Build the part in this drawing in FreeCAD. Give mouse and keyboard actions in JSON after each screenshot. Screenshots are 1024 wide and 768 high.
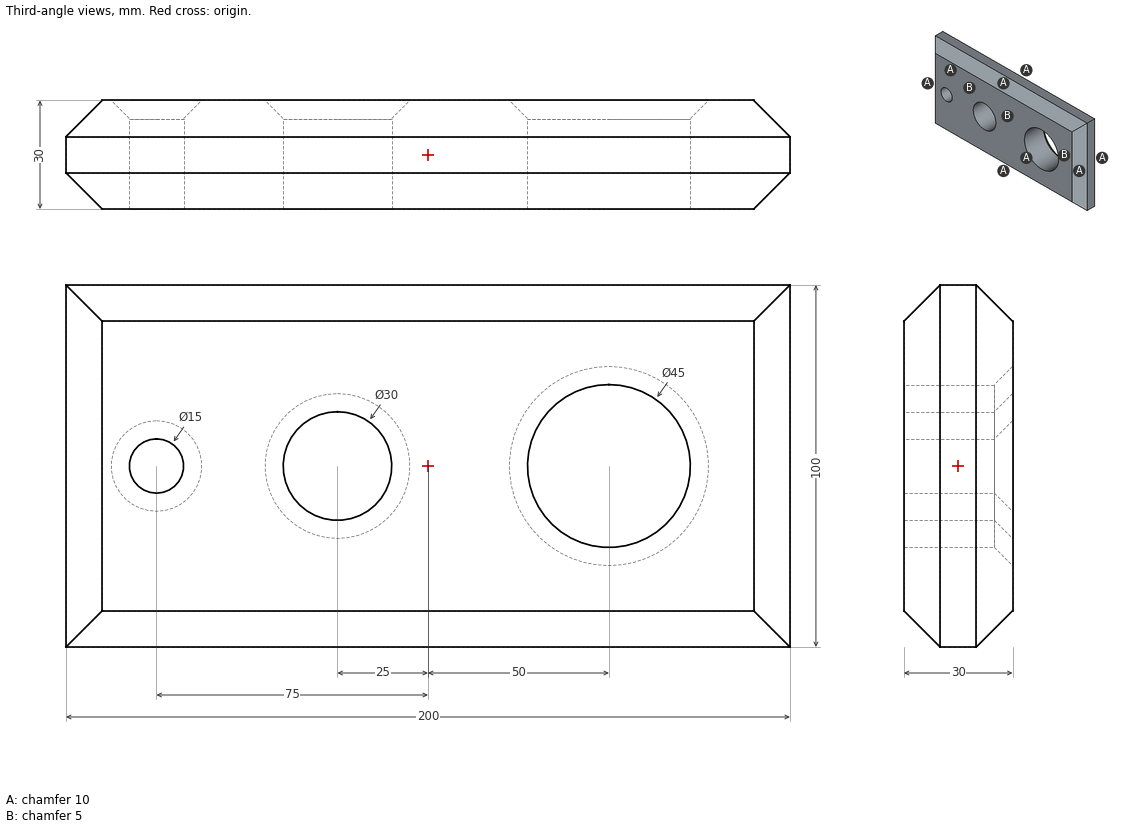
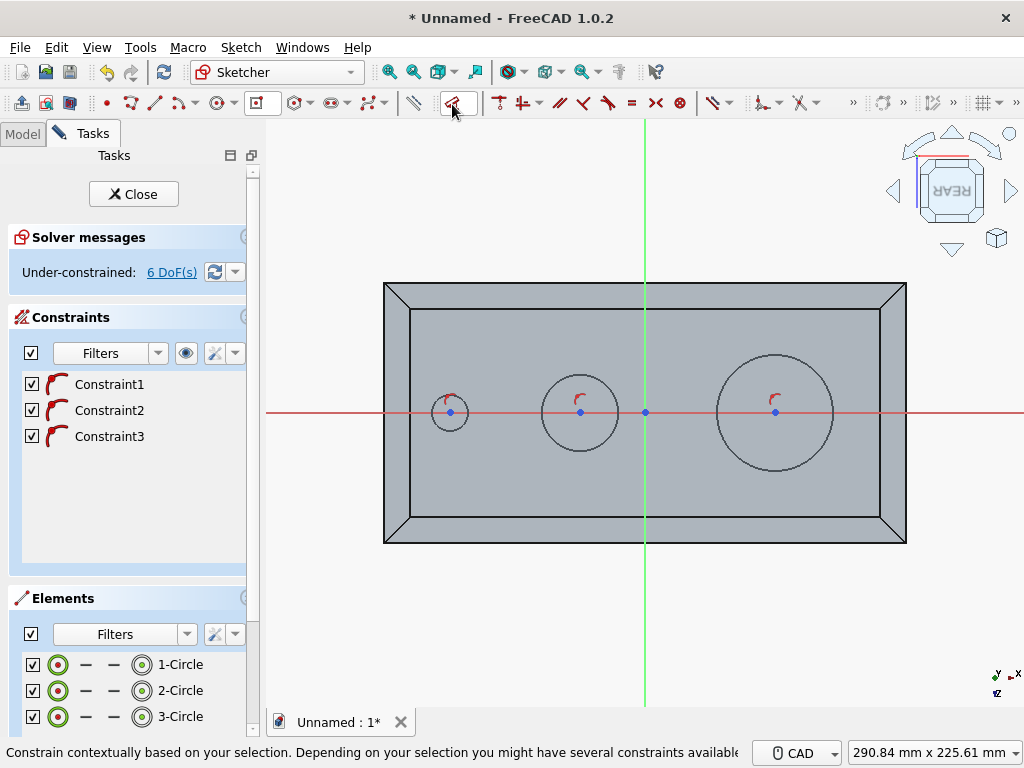
{"action": "left_click", "coordinate": [463, 400]}
{"action": "left_click", "coordinate": [486, 377]}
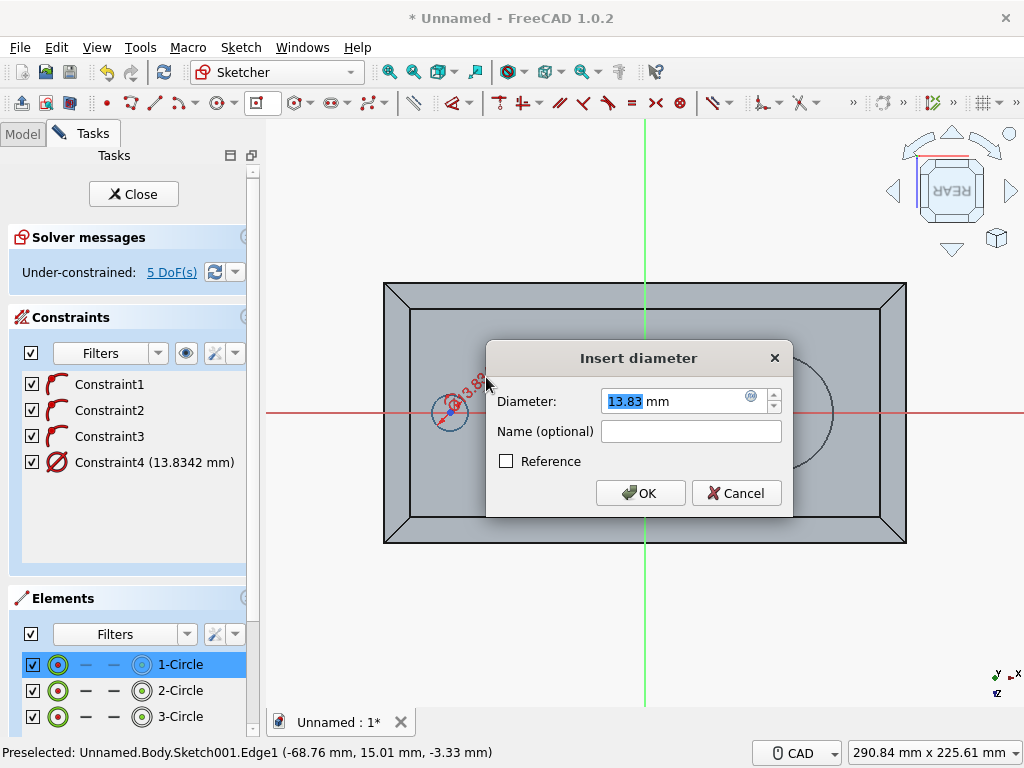
{"action": "type", "text": "15"}
{"action": "key", "text": "Return"}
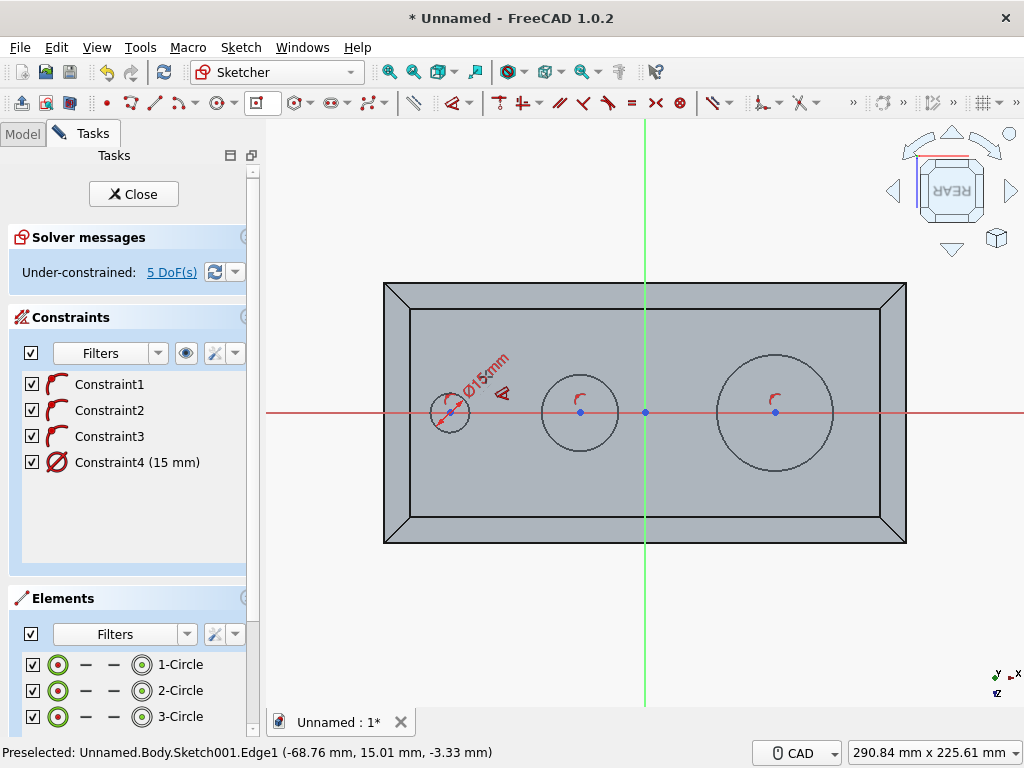
{"action": "left_click", "coordinate": [607, 386]}
{"action": "left_click", "coordinate": [630, 363]}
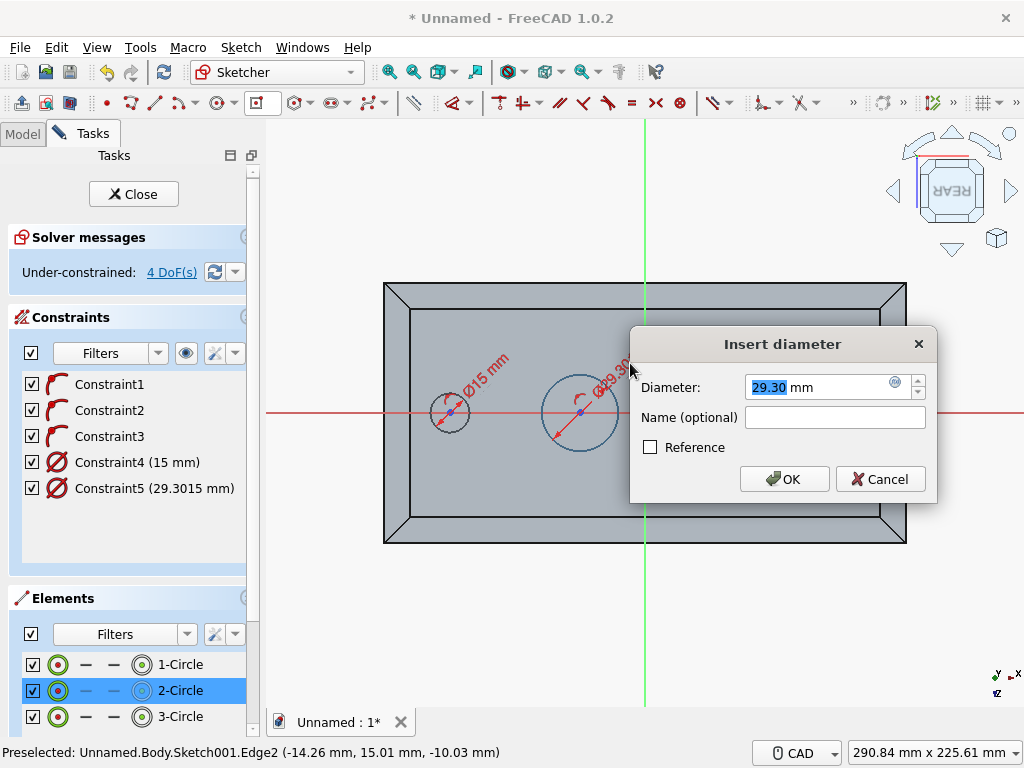
{"action": "type", "text": "30"}
{"action": "key", "text": "Return"}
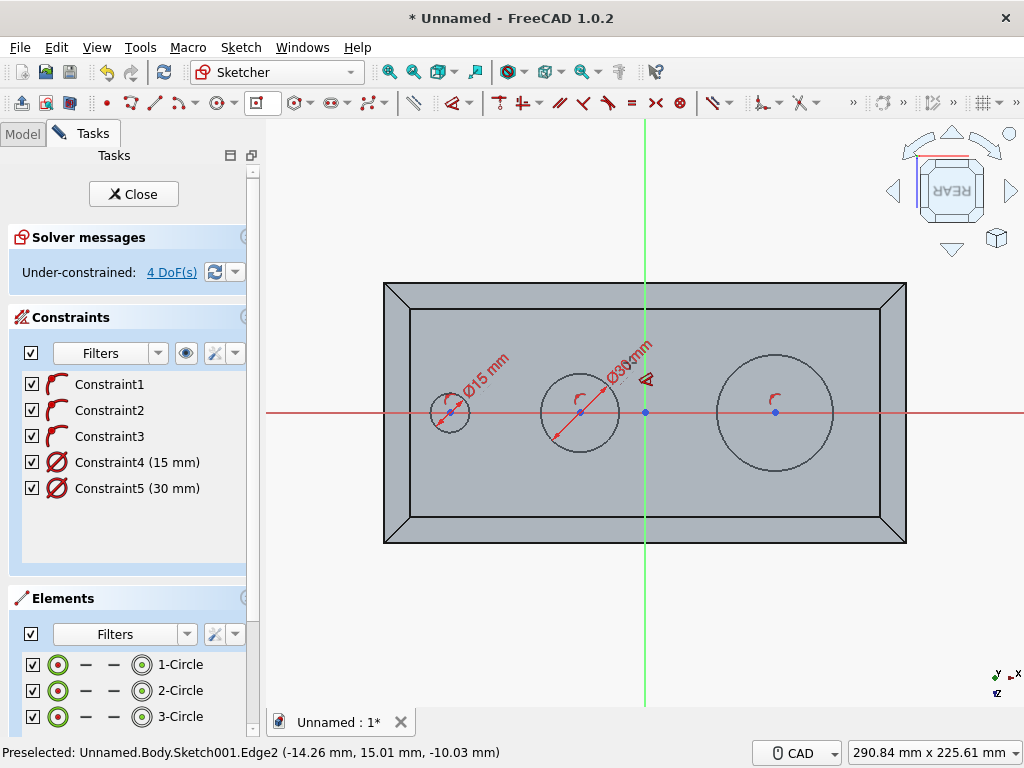
{"action": "left_click", "coordinate": [816, 372]}
{"action": "left_click", "coordinate": [839, 349]}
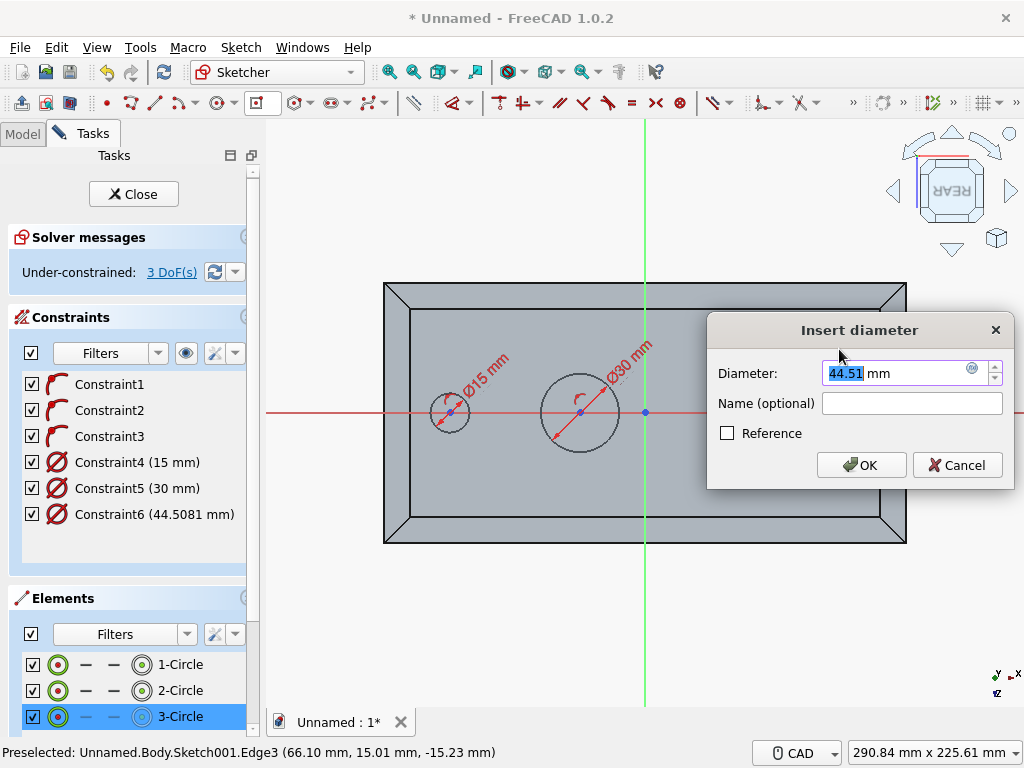
{"action": "type", "text": "45"}
{"action": "key", "text": "Return"}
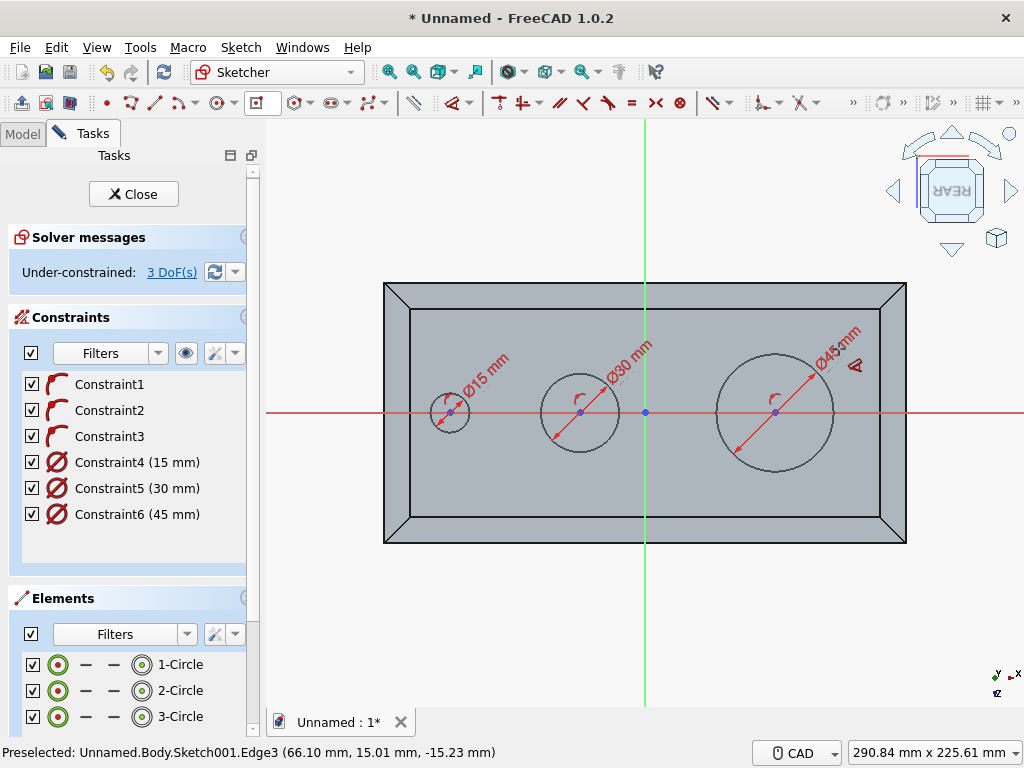
{"action": "left_click", "coordinate": [450, 413]}
{"action": "left_click", "coordinate": [503, 447]}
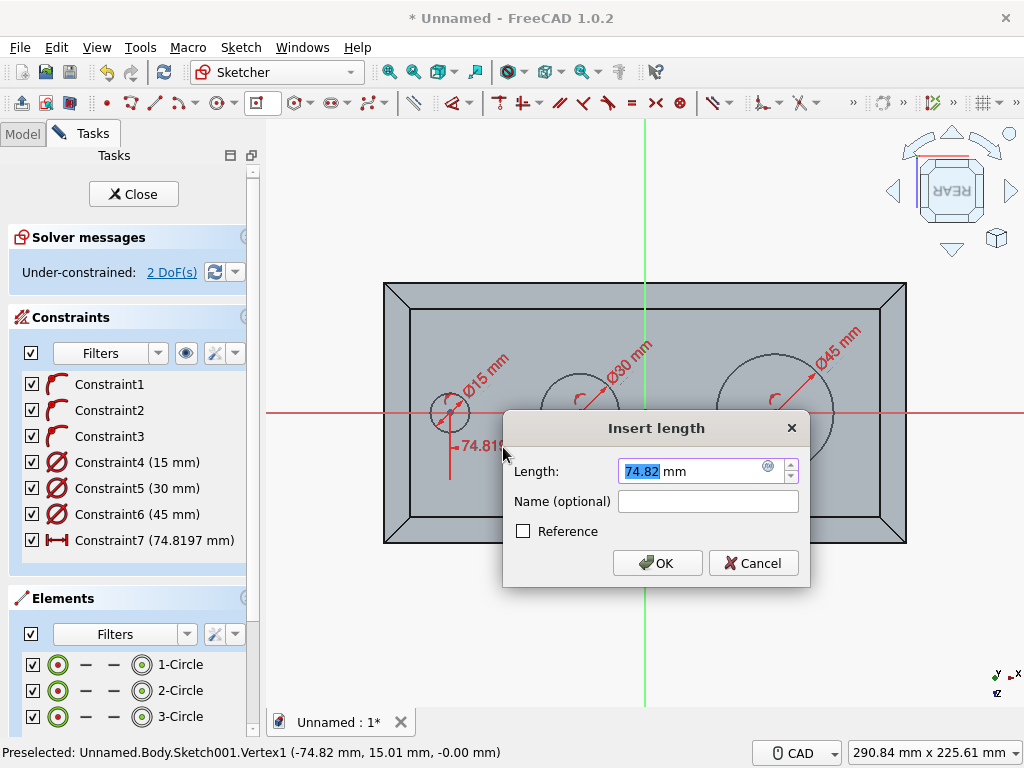
{"action": "type", "text": "75"}
{"action": "key", "text": "Return"}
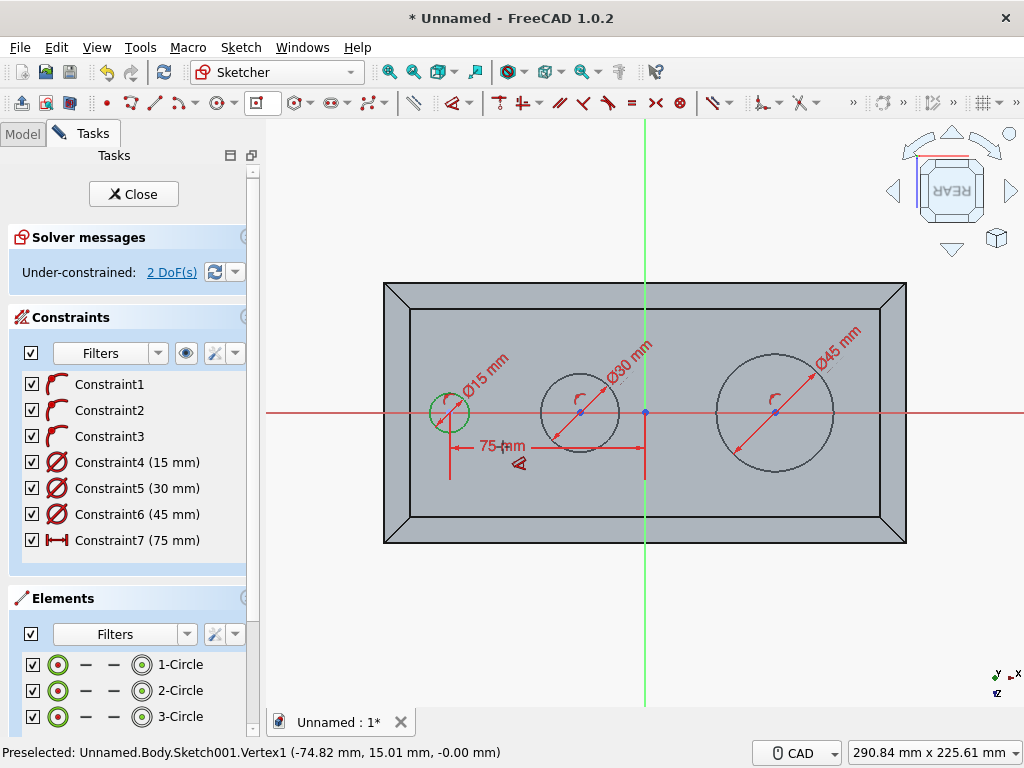
{"action": "left_click", "coordinate": [580, 413]}
{"action": "left_click", "coordinate": [627, 447]}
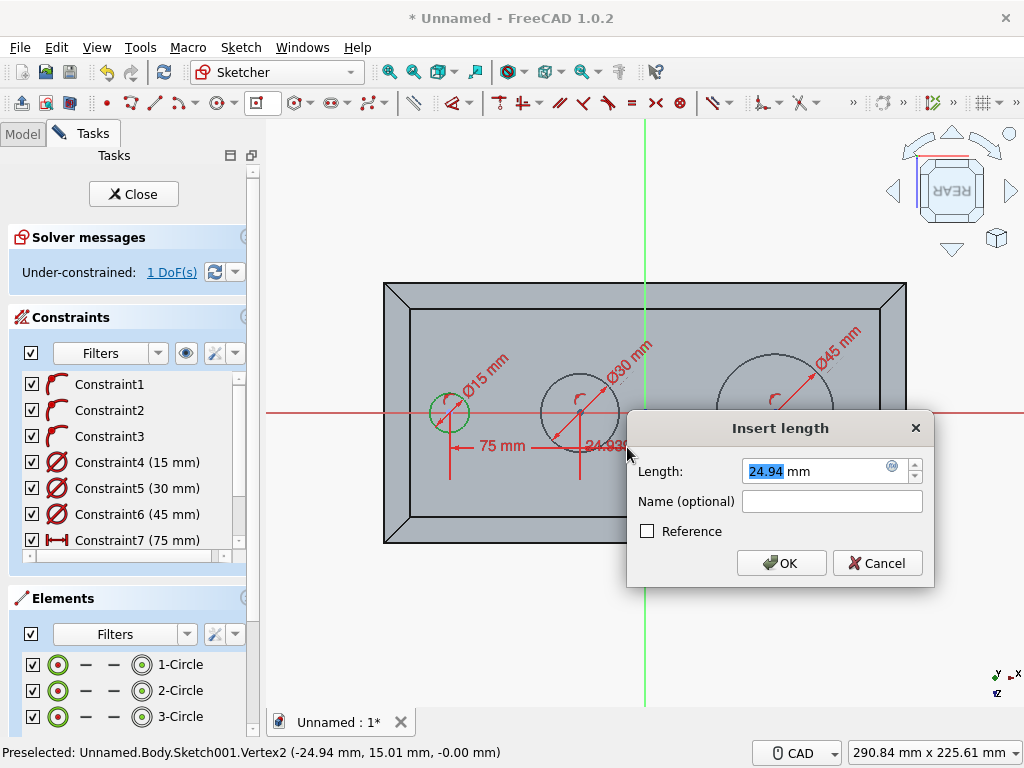
{"action": "type", "text": "25"}
{"action": "key", "text": "Return"}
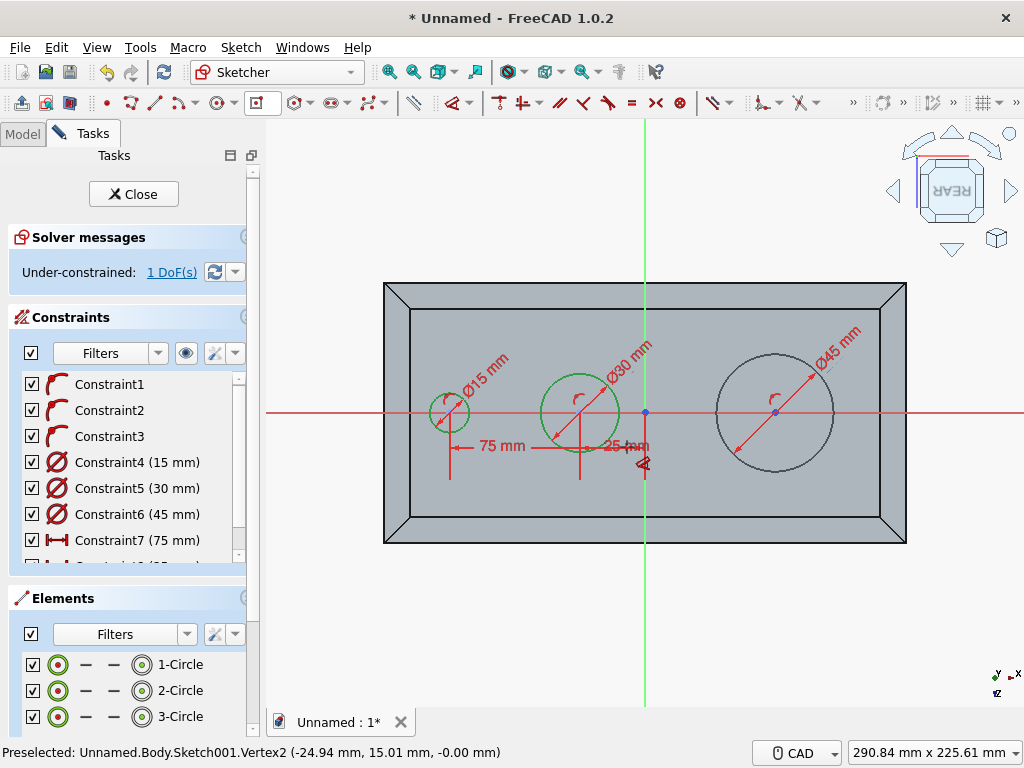
{"action": "left_click", "coordinate": [775, 413]}
{"action": "left_click", "coordinate": [710, 447]}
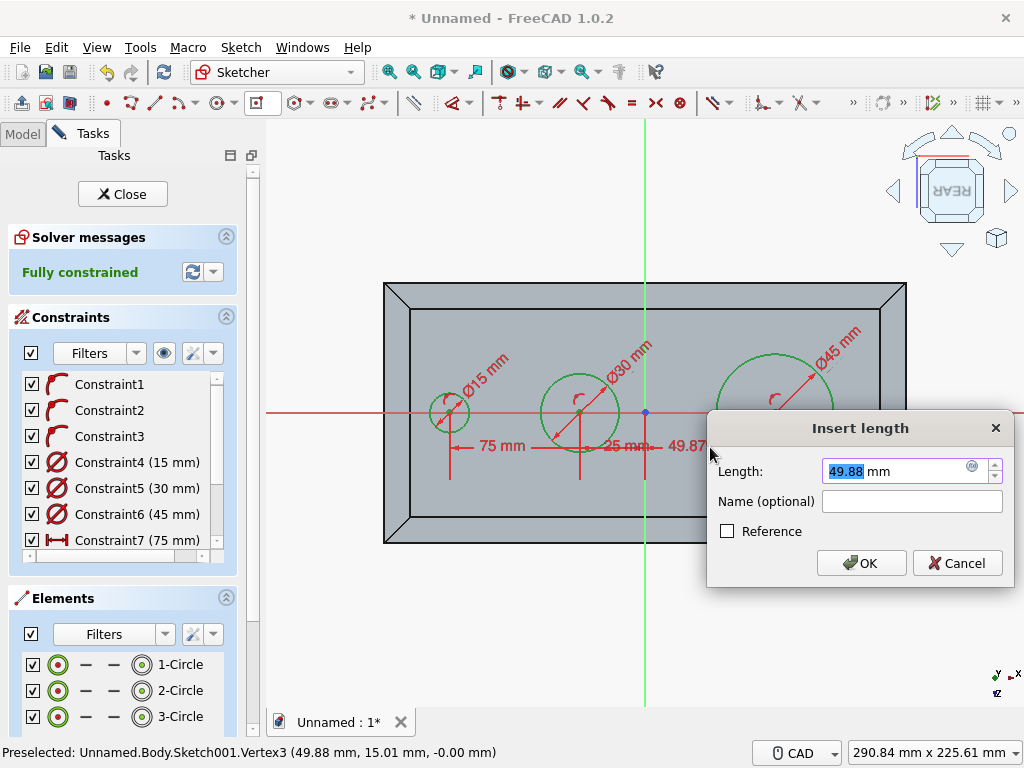
{"action": "type", "text": "50"}
{"action": "key", "text": "Return"}
{"action": "key", "text": "Escape"}